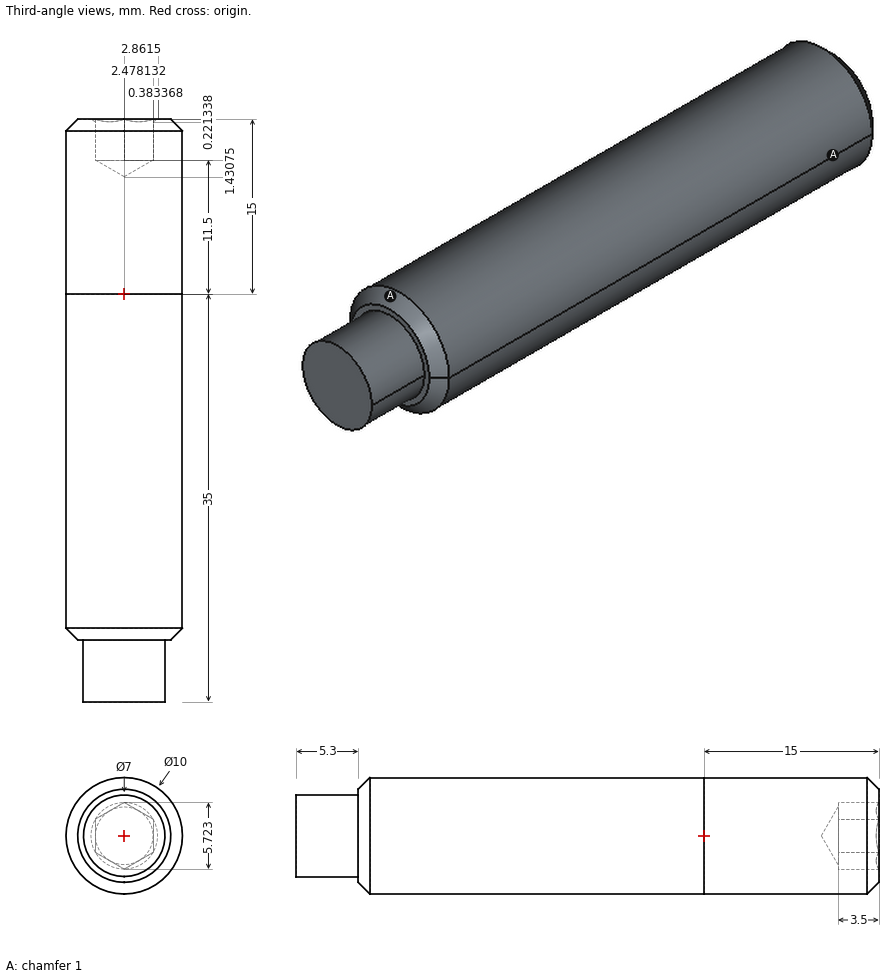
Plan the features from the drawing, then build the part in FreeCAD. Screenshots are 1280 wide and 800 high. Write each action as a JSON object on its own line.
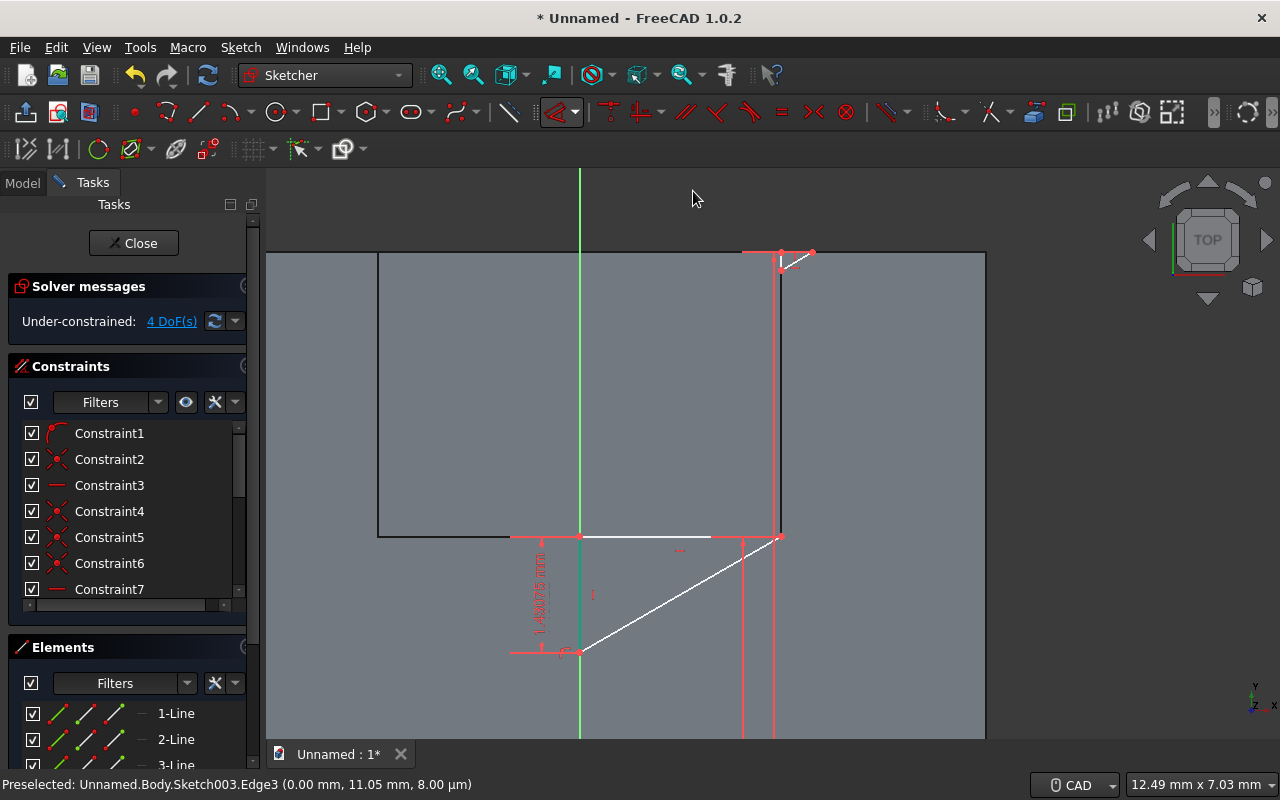
{"action": "left_click", "coordinate": [812, 252]}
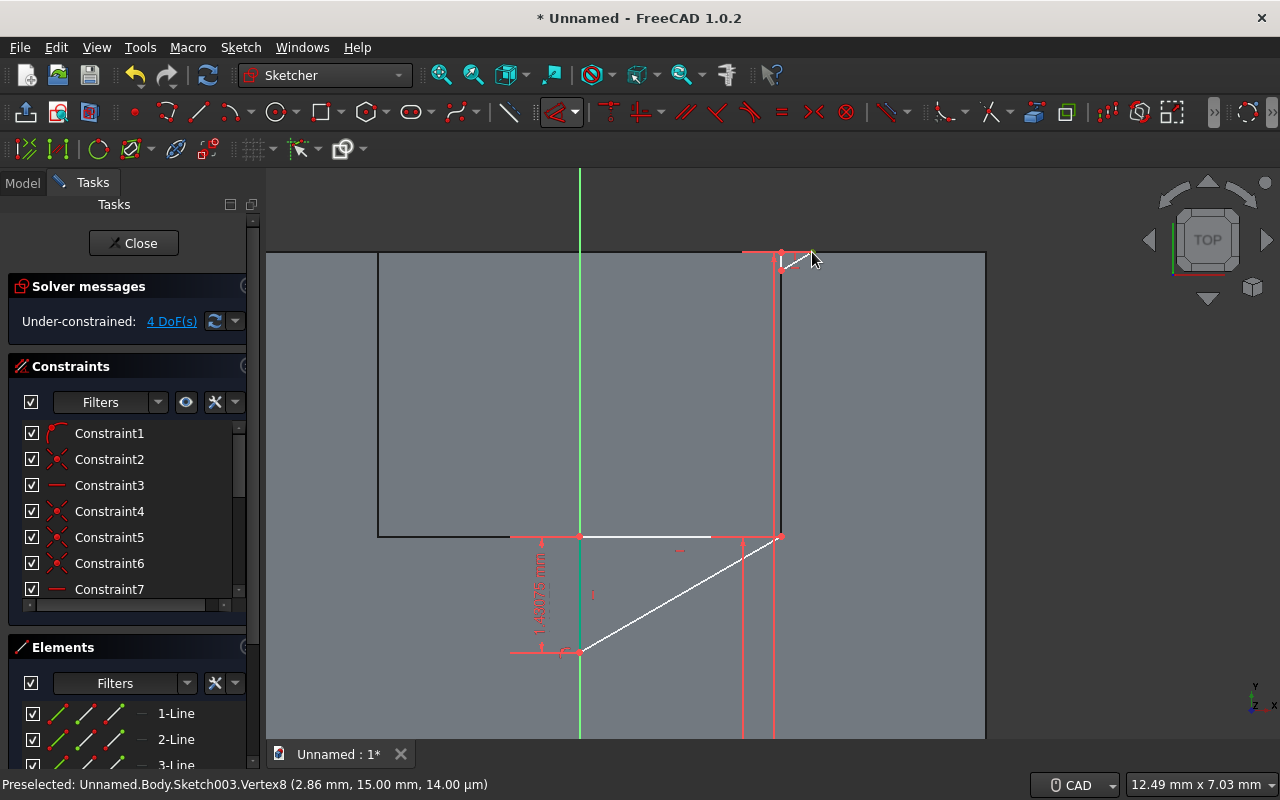
{"action": "key", "text": "l"}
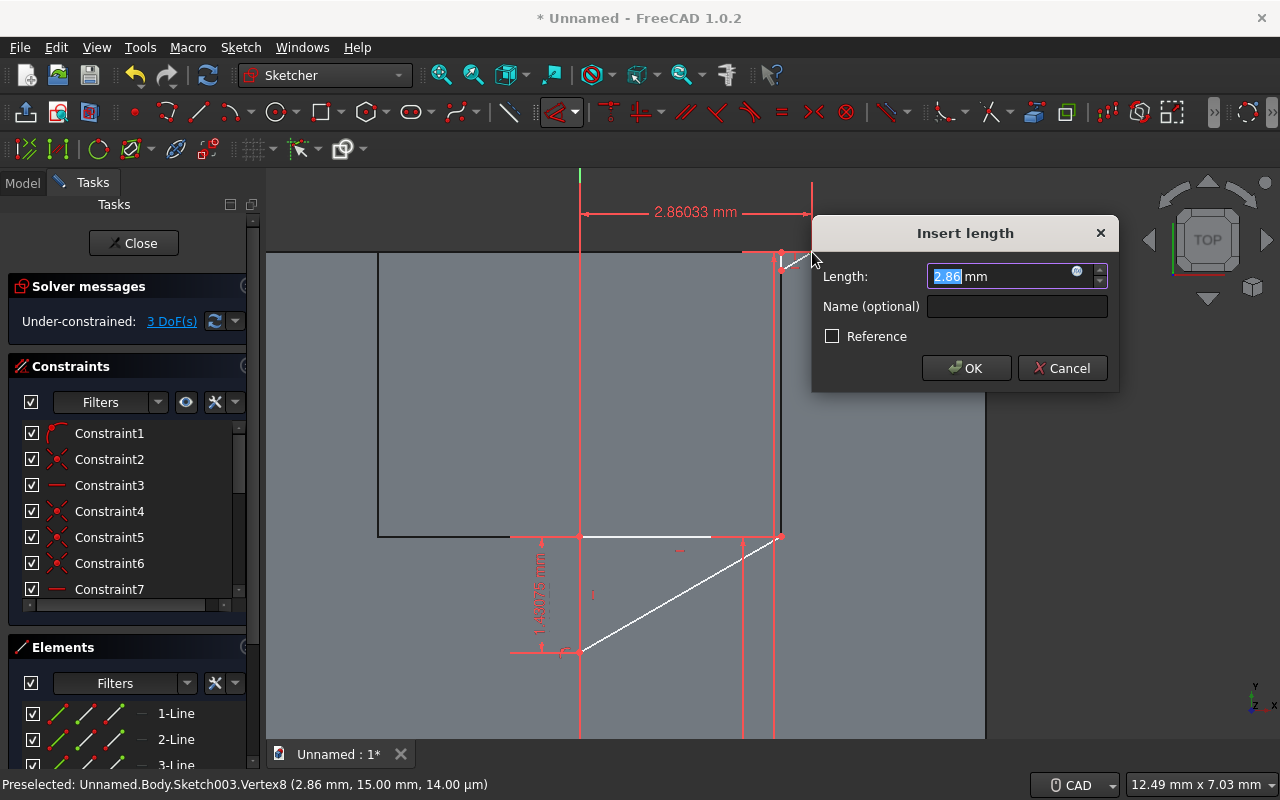
{"action": "type", "text": "2.8615"}
{"action": "key", "text": "Return"}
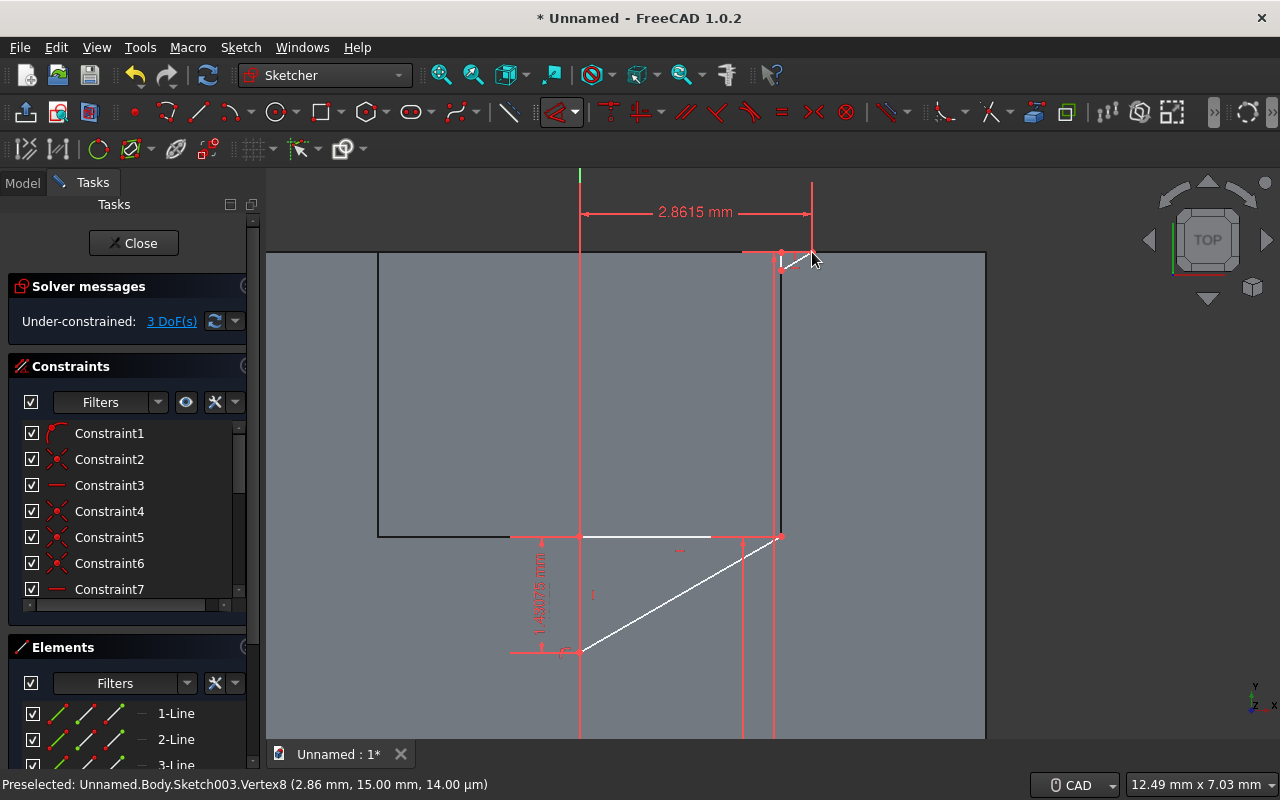
{"action": "left_click", "coordinate": [721, 537]}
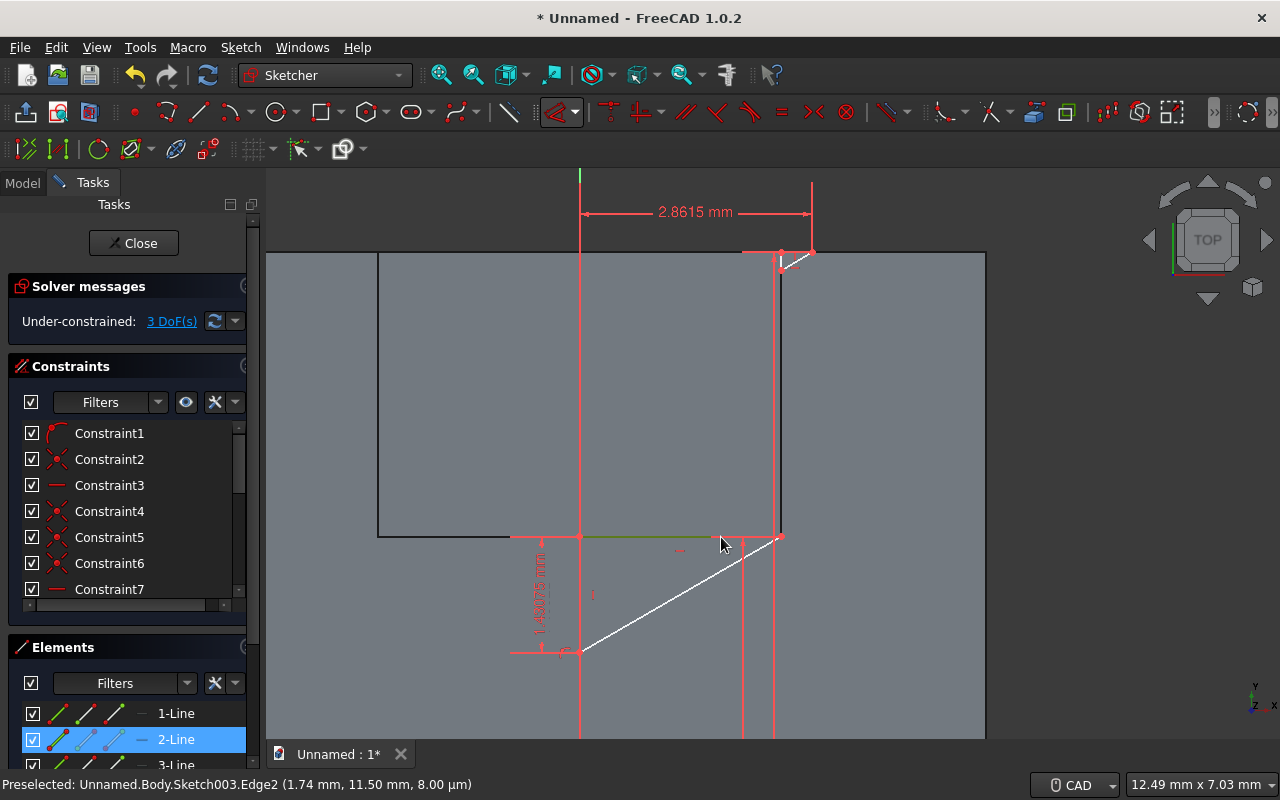
{"action": "left_click", "coordinate": [578, 112]}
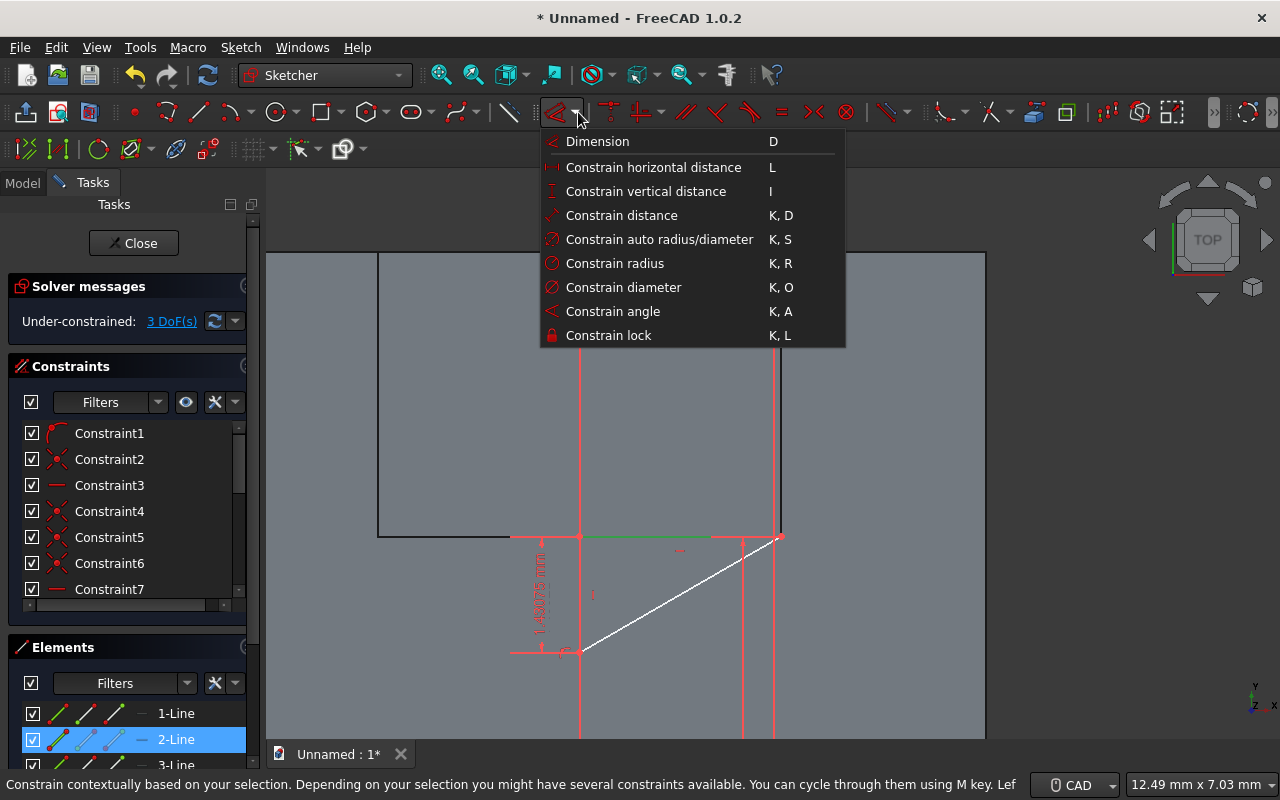
{"action": "left_click", "coordinate": [693, 167]}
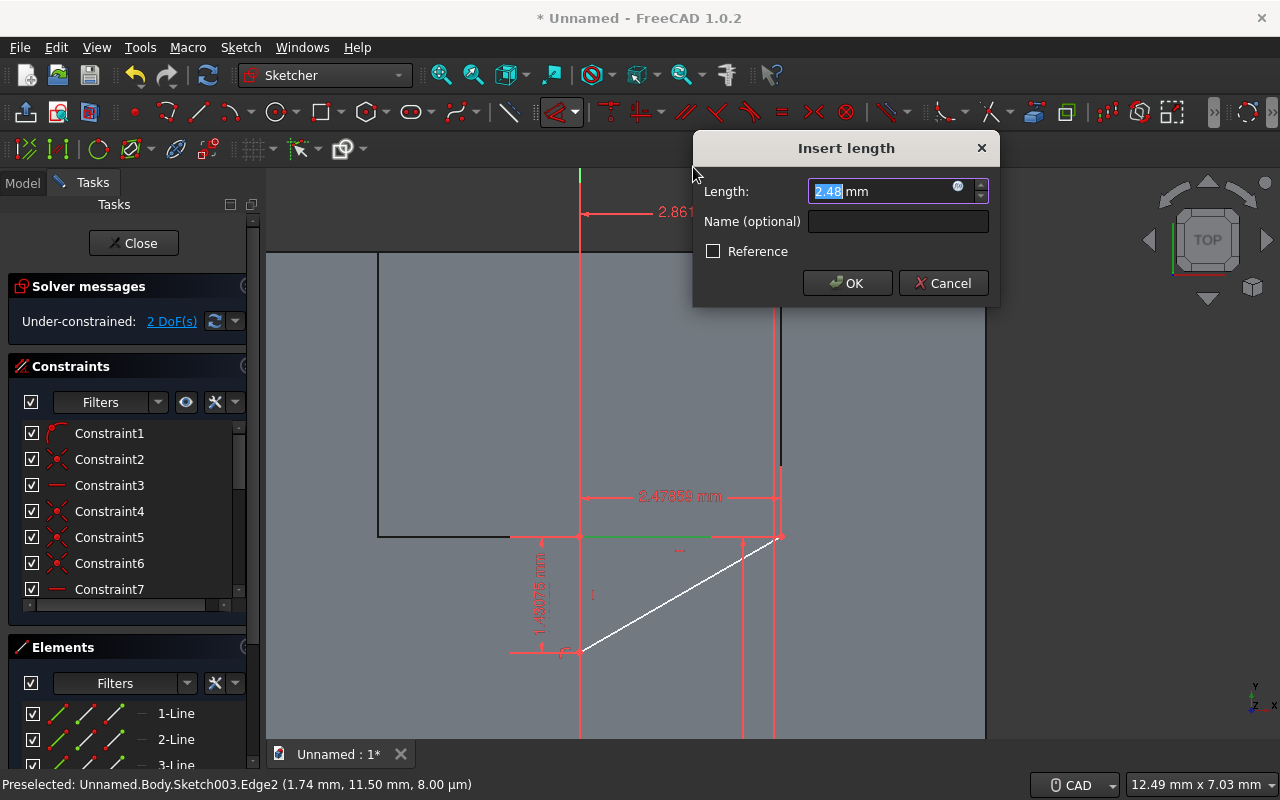
{"action": "type", "text": "2.478132"}
{"action": "key", "text": "Return"}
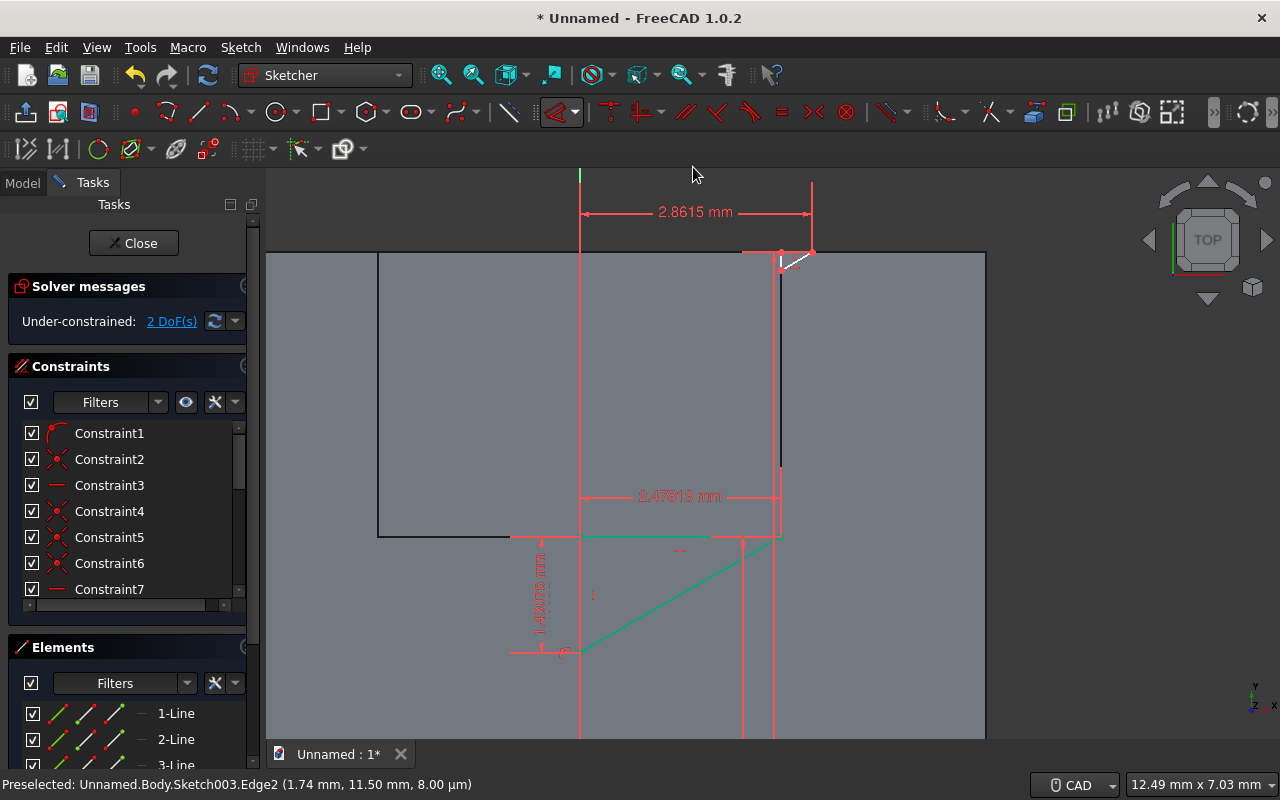
{"action": "scroll", "coordinate": [790, 252], "scroll_direction": "up", "scroll_amount": 2}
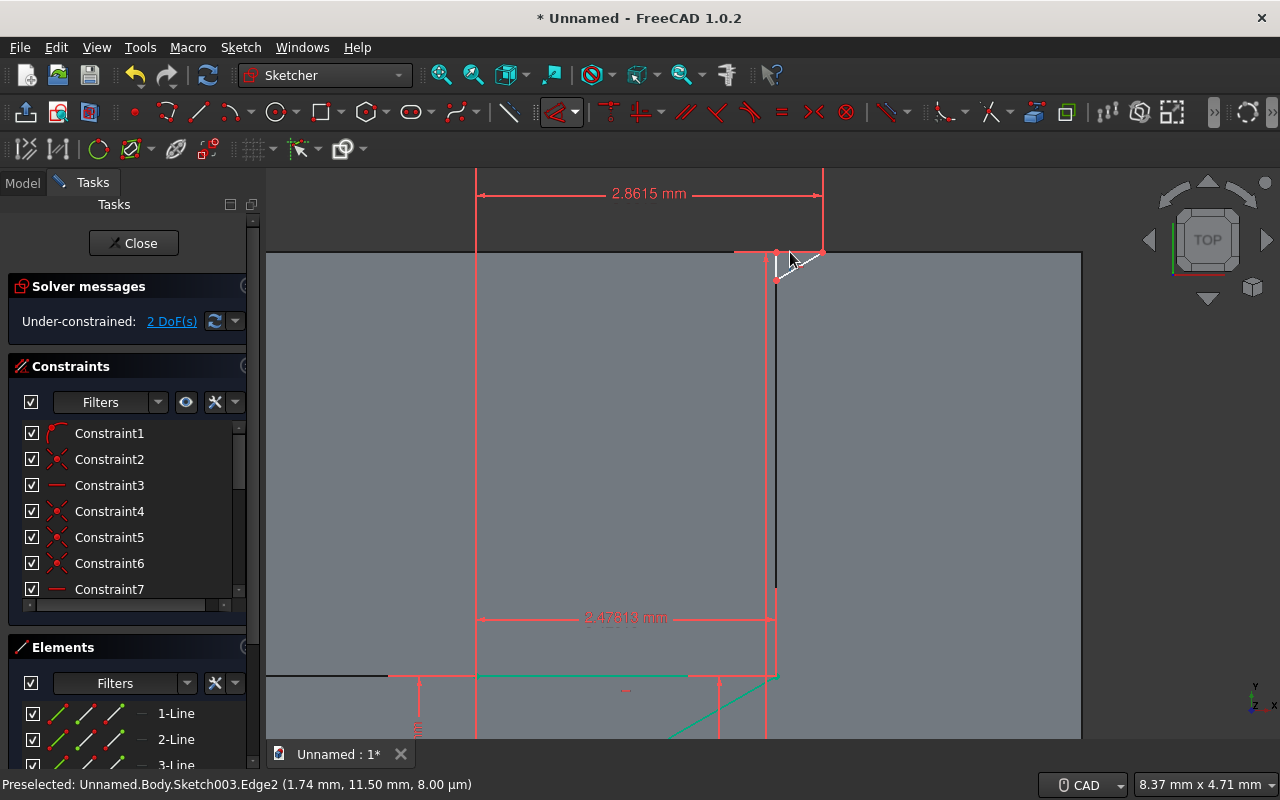
{"action": "left_click", "coordinate": [790, 252]}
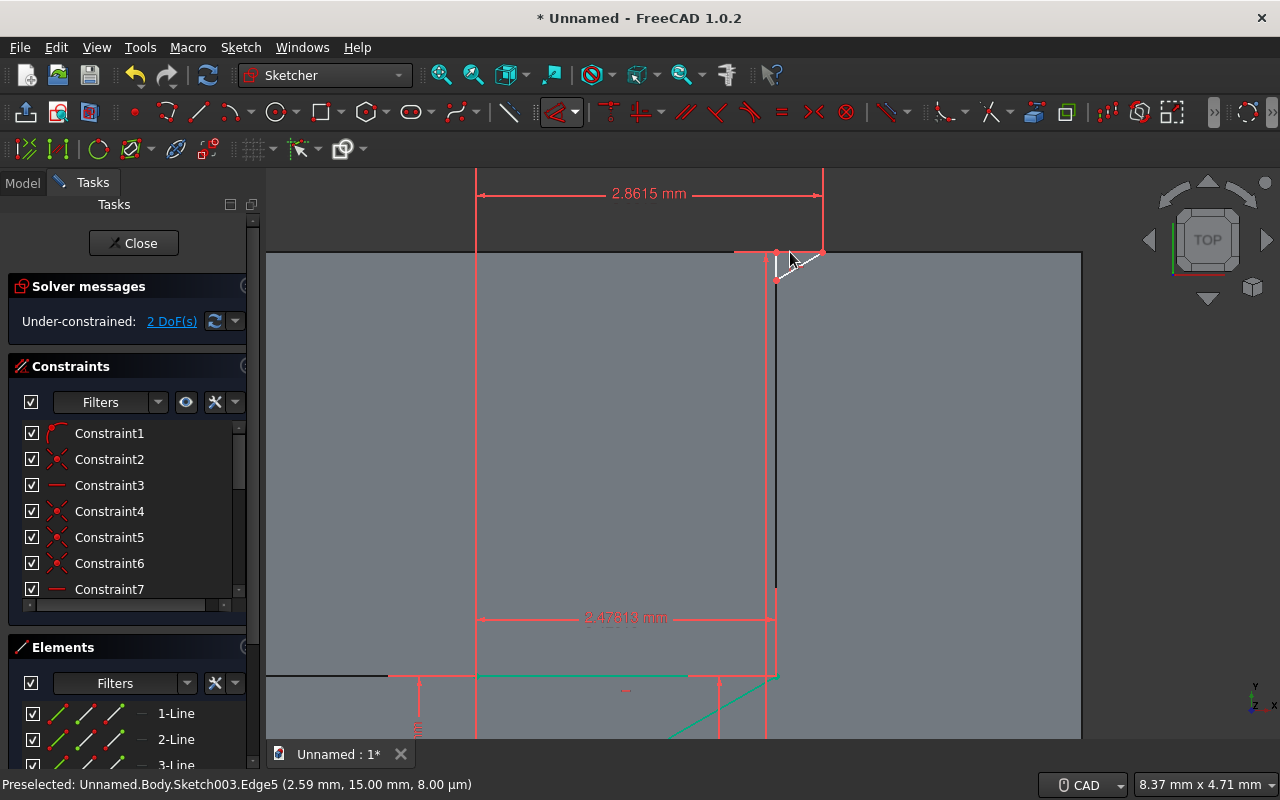
{"action": "left_click", "coordinate": [578, 112]}